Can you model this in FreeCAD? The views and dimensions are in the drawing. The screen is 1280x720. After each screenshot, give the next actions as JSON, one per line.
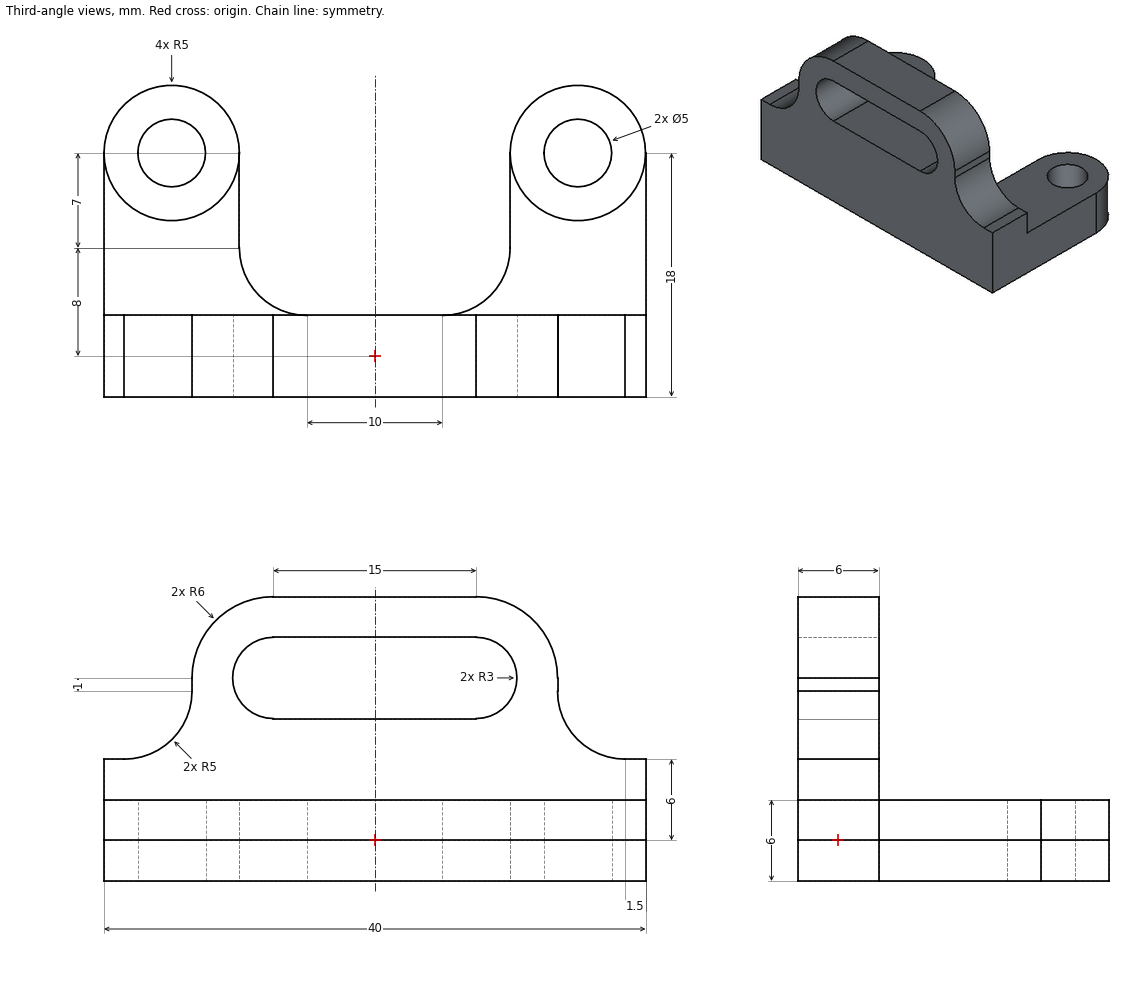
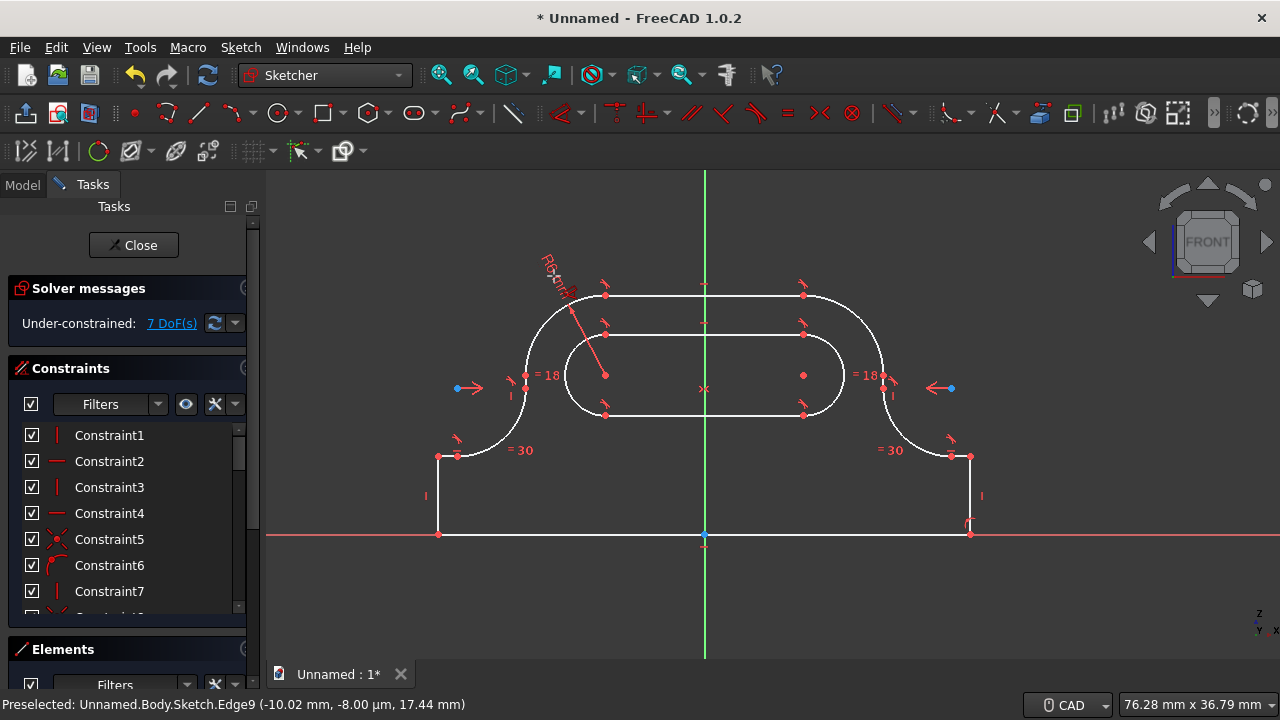
{"action": "left_click", "coordinate": [891, 419]}
{"action": "left_click", "coordinate": [862, 433]}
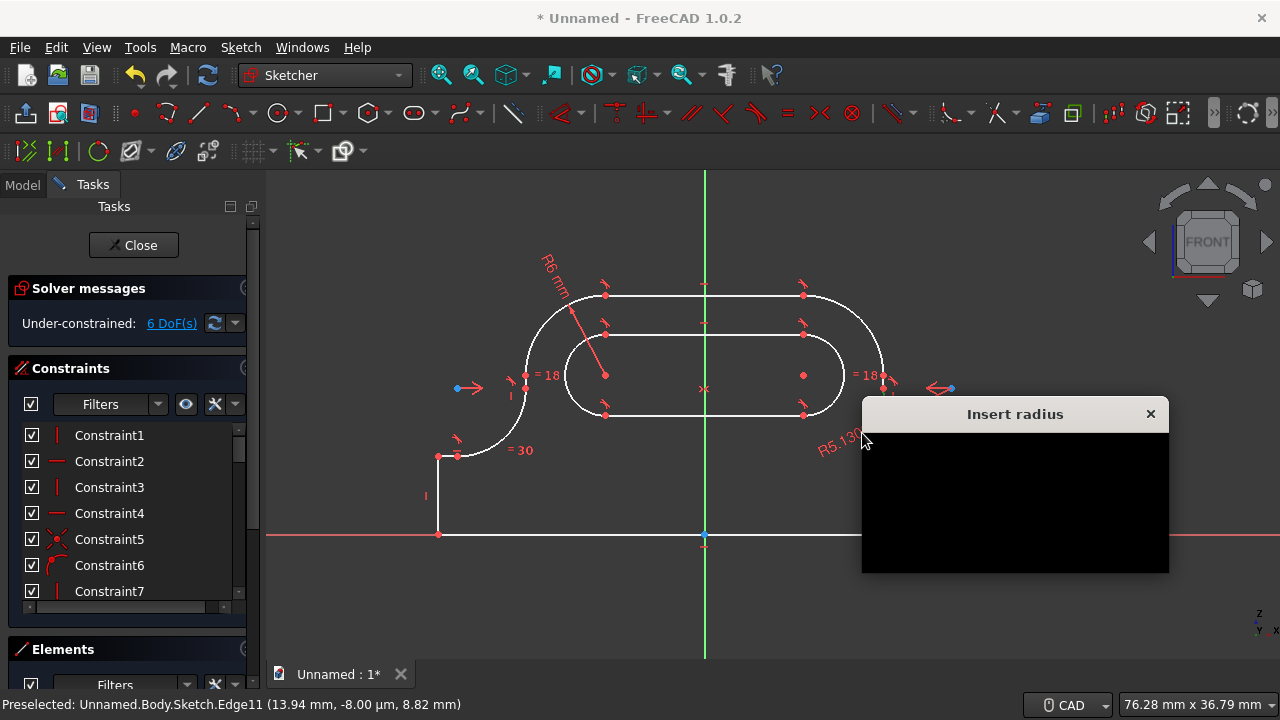
{"action": "type", "text": "5"}
{"action": "key", "text": "Return"}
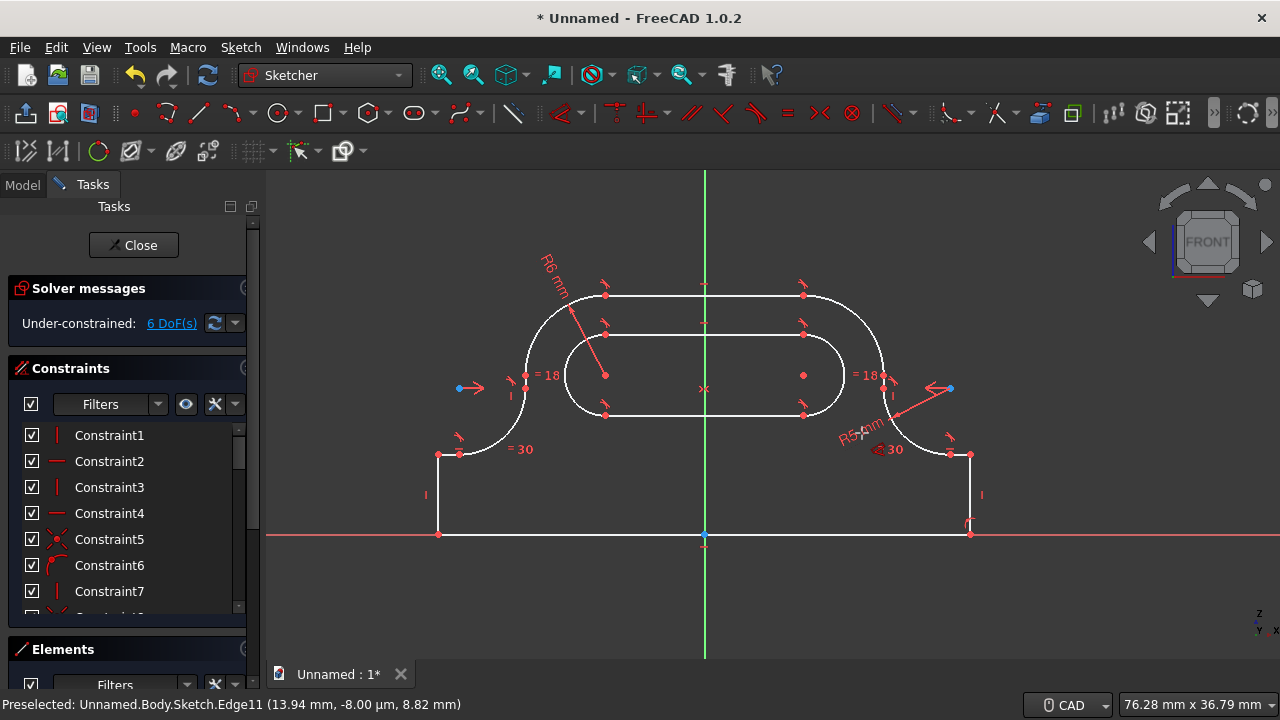
{"action": "left_click", "coordinate": [573, 352]}
{"action": "left_click", "coordinate": [538, 402]}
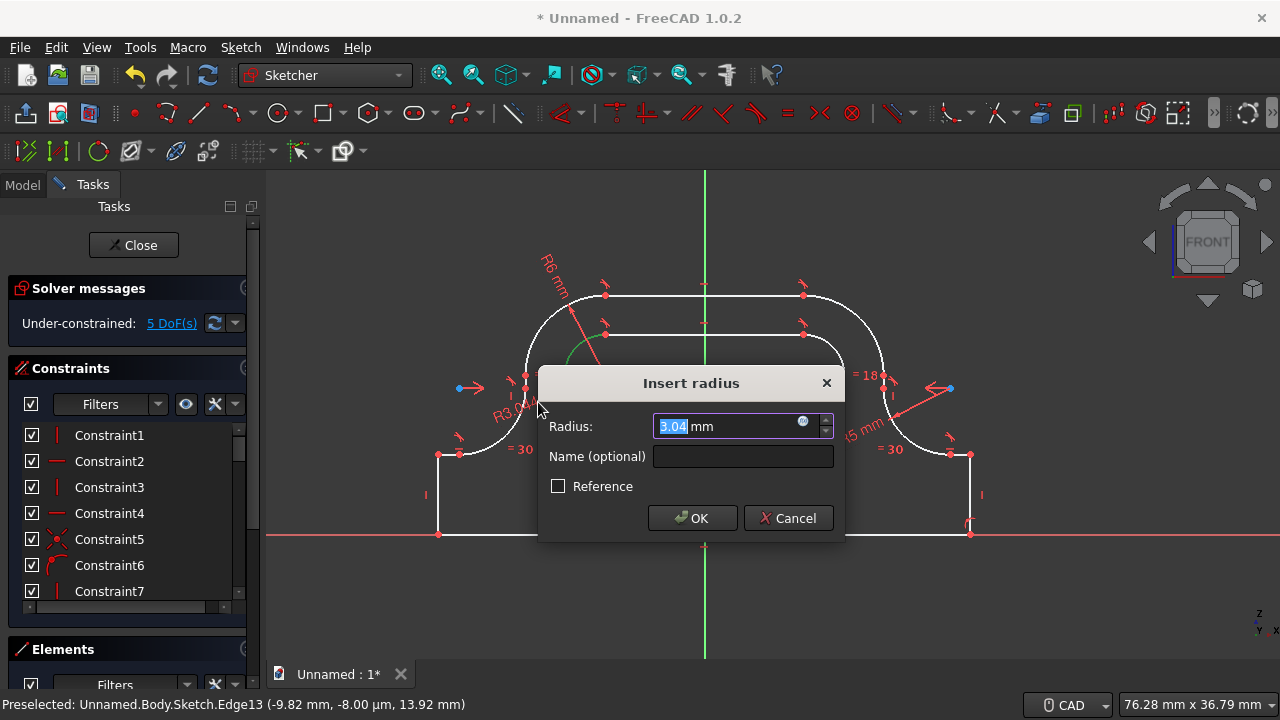
{"action": "type", "text": "3"}
{"action": "key", "text": "Return"}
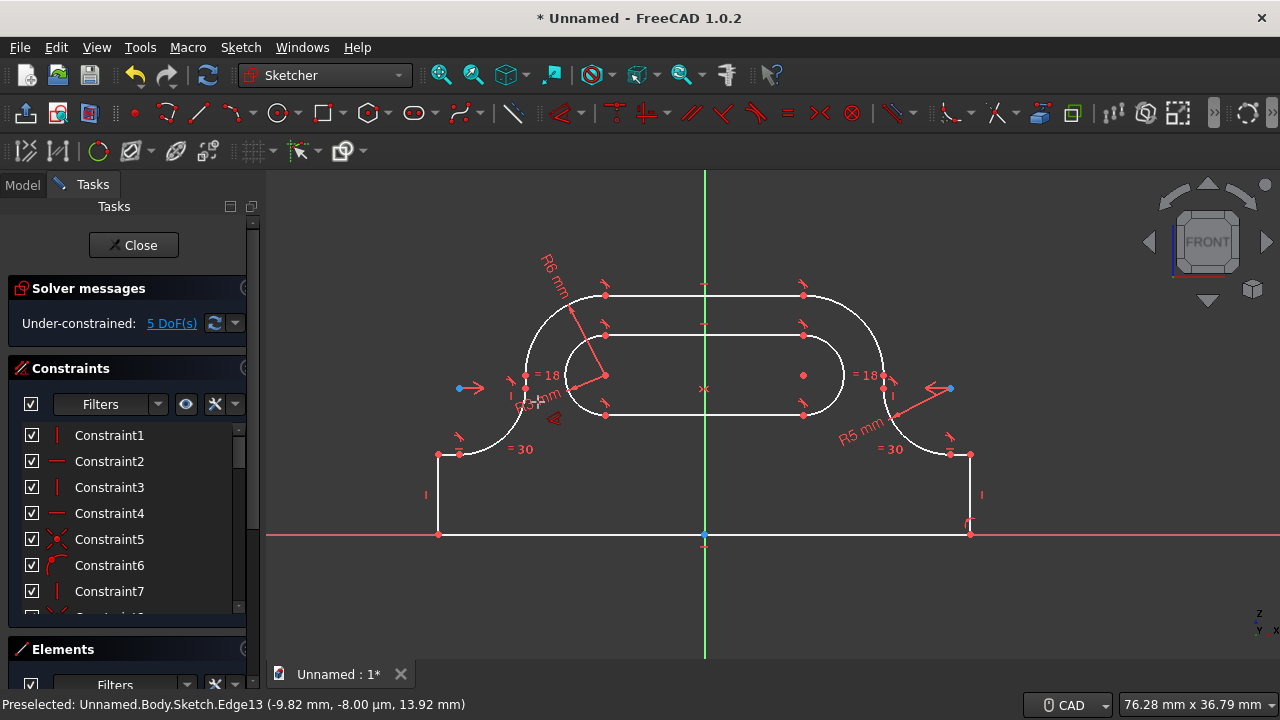
{"action": "scroll", "coordinate": [526, 382], "scroll_direction": "up", "scroll_amount": 6}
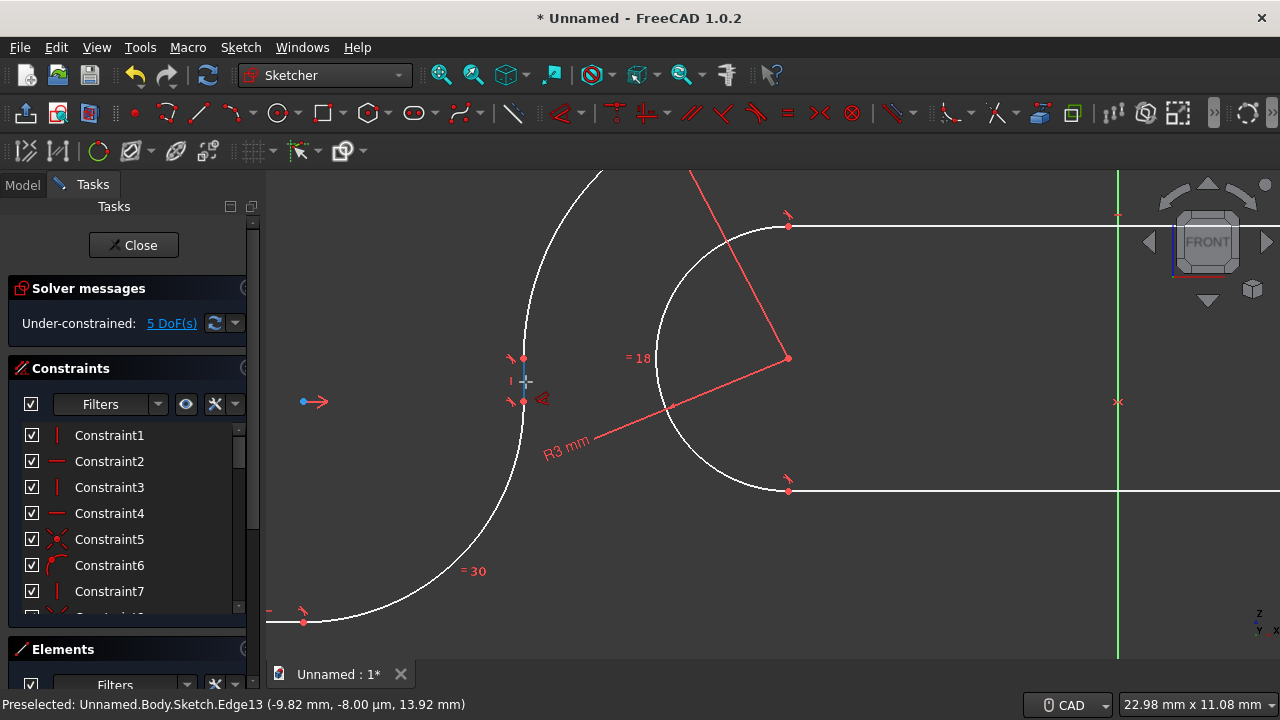
{"action": "left_click", "coordinate": [524, 380]}
{"action": "left_click", "coordinate": [490, 380]}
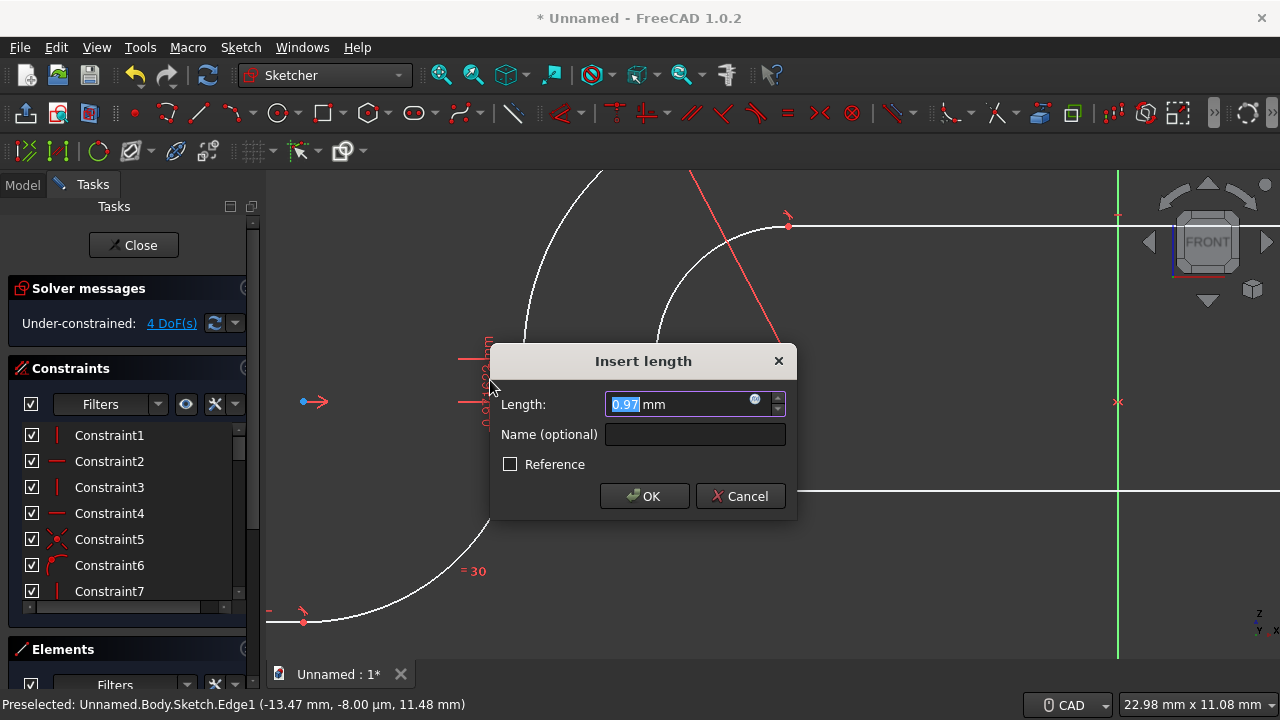
{"action": "type", "text": "1"}
{"action": "key", "text": "Return"}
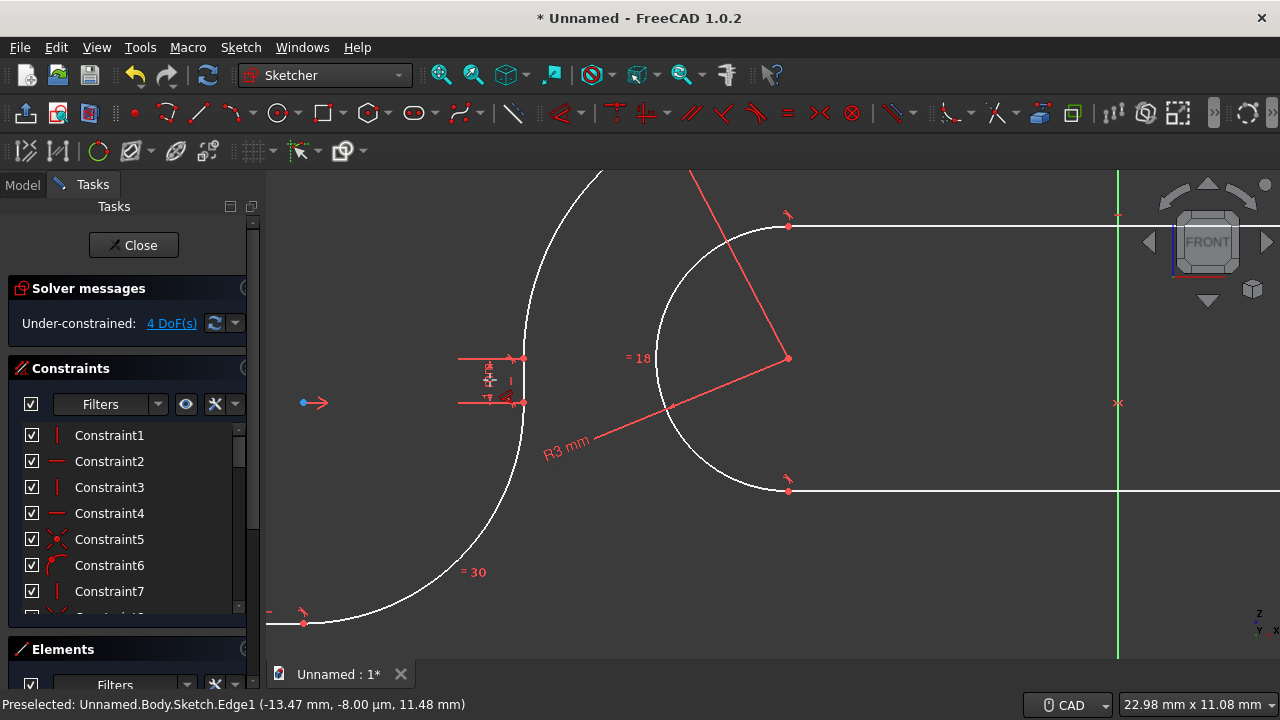
{"action": "scroll", "coordinate": [526, 382], "scroll_direction": "down", "scroll_amount": 6}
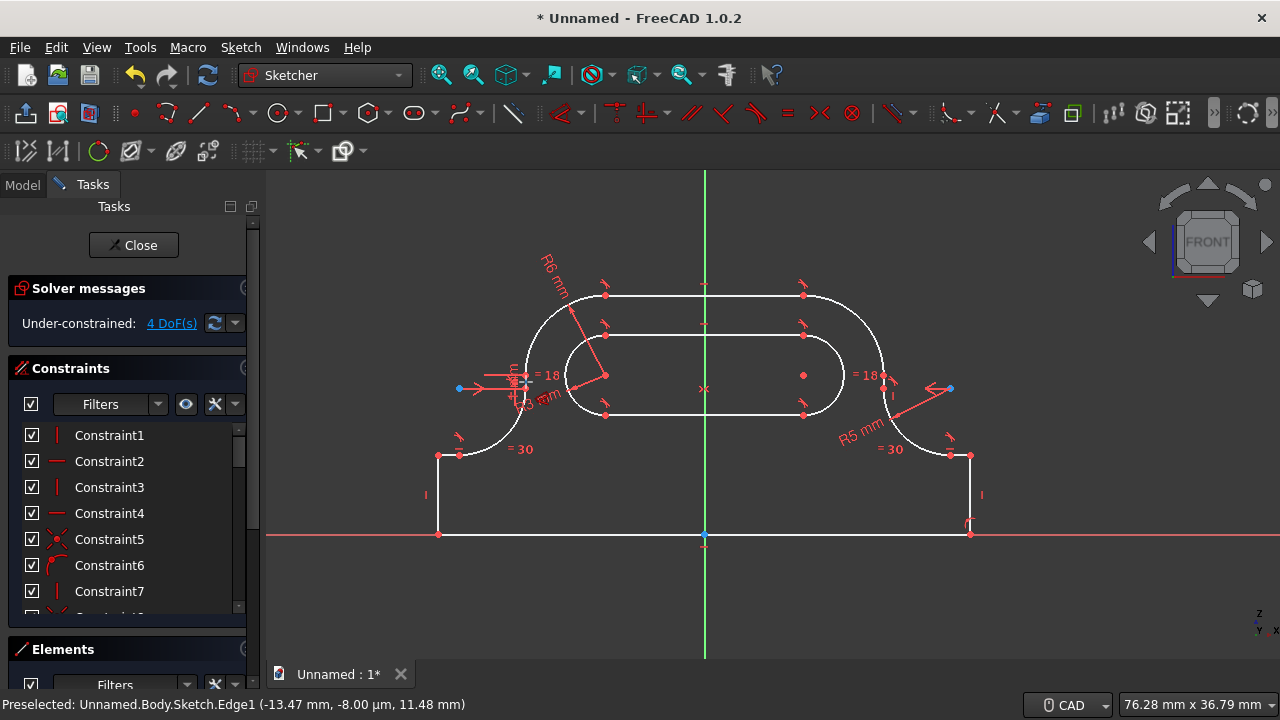
{"action": "left_click", "coordinate": [970, 479]}
{"action": "left_click", "coordinate": [1004, 495]}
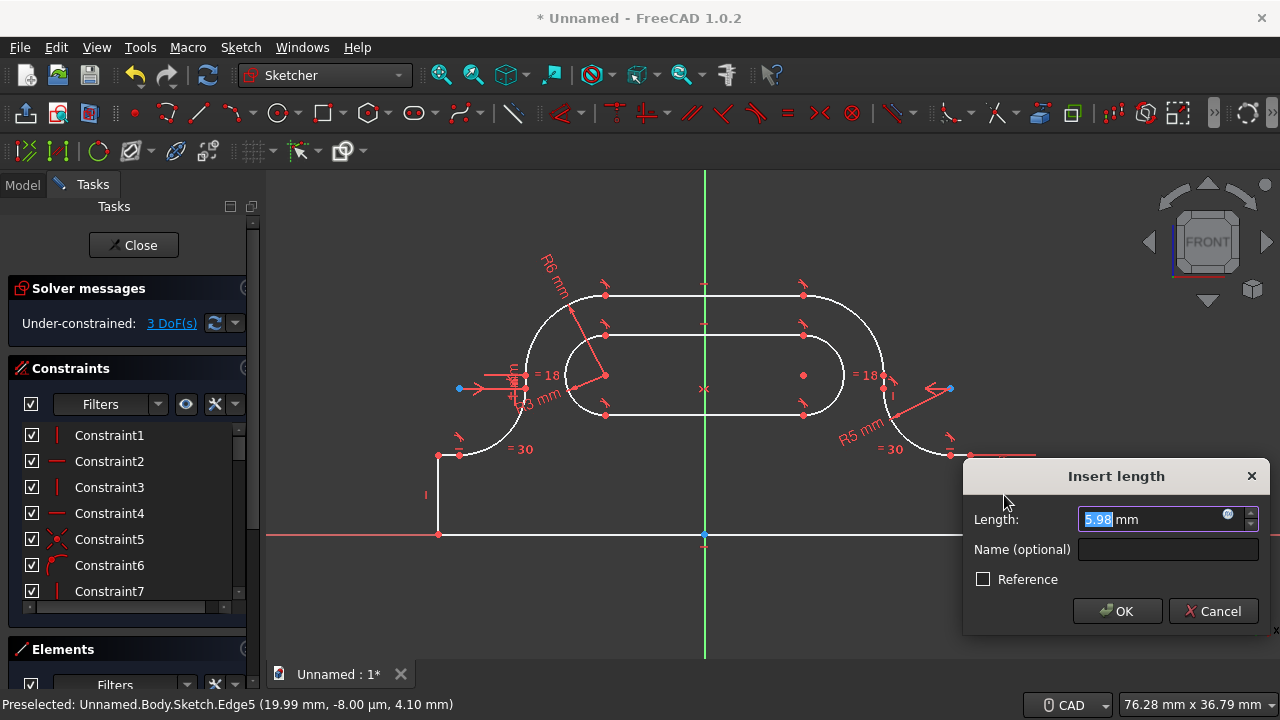
{"action": "type", "text": "6"}
{"action": "key", "text": "Return"}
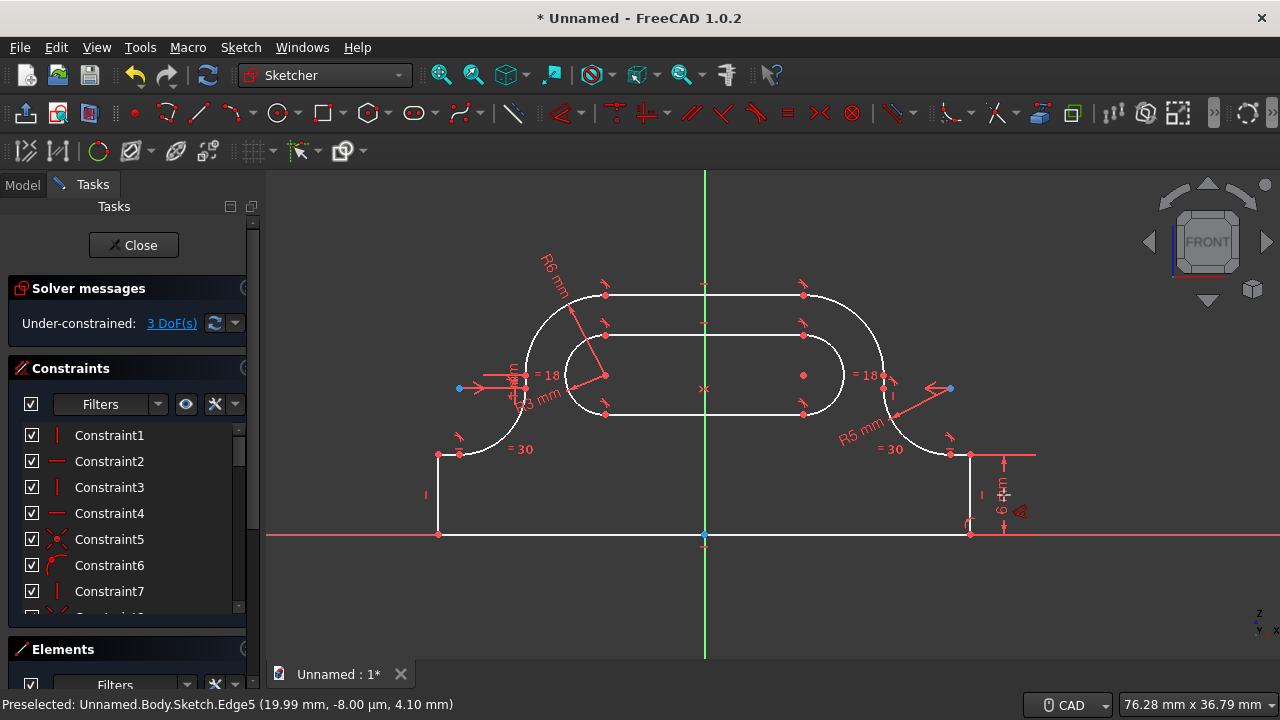
{"action": "left_click", "coordinate": [665, 295]}
{"action": "left_click", "coordinate": [659, 261]}